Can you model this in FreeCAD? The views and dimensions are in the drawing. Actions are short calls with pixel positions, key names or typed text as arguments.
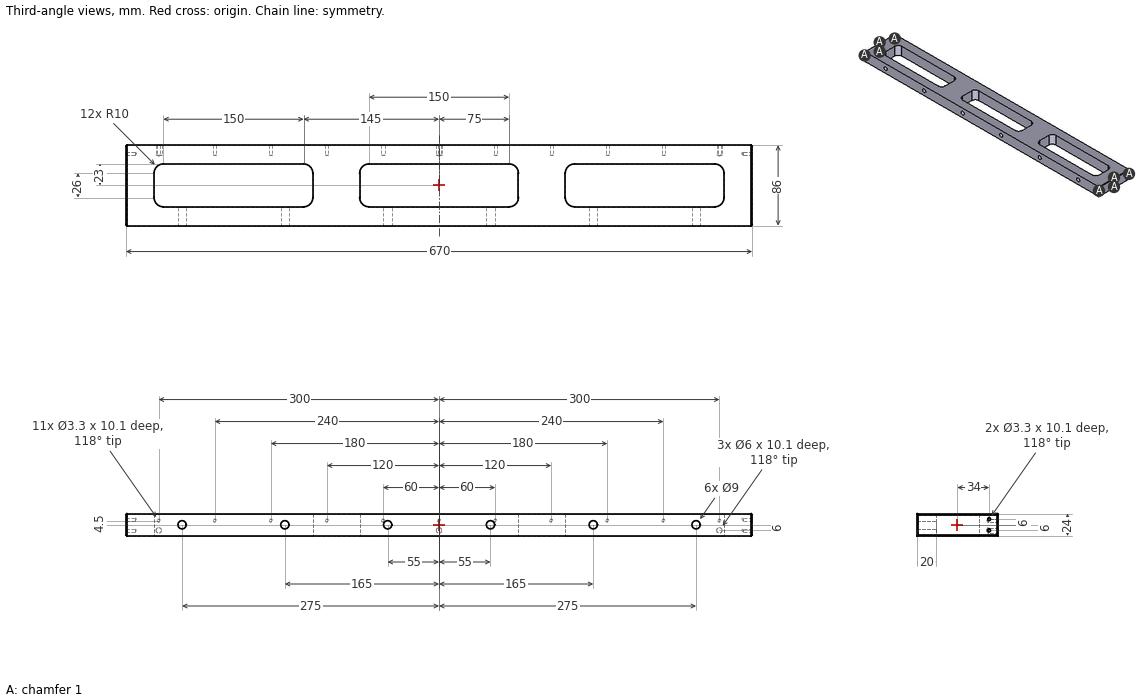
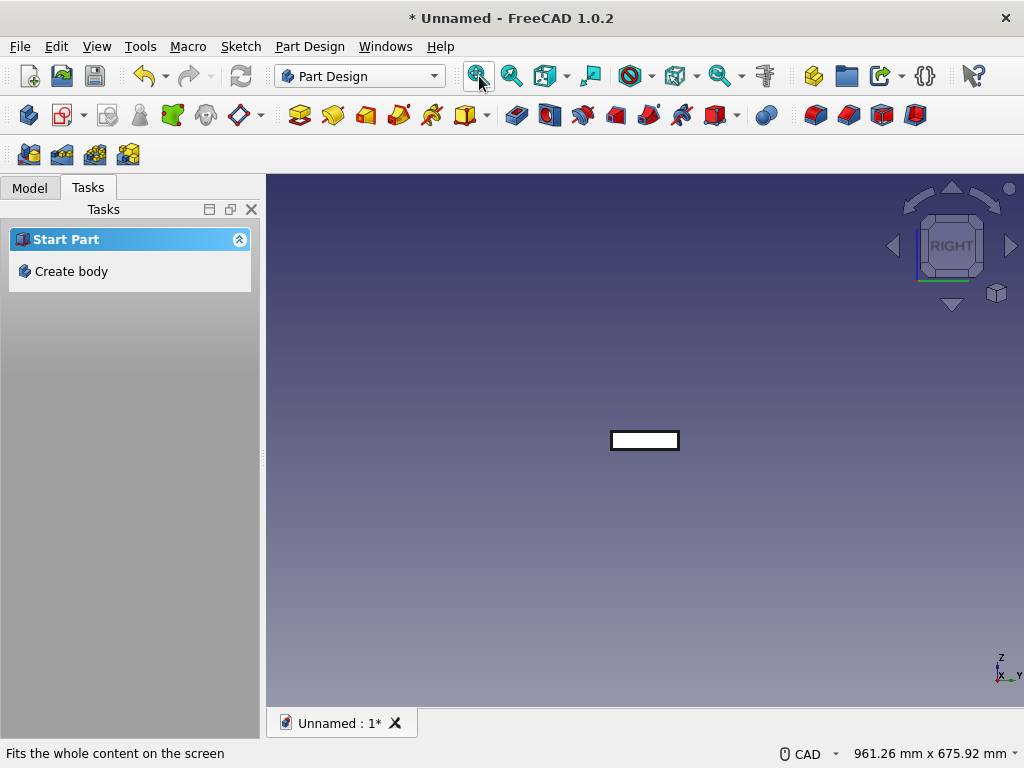
click(664, 439)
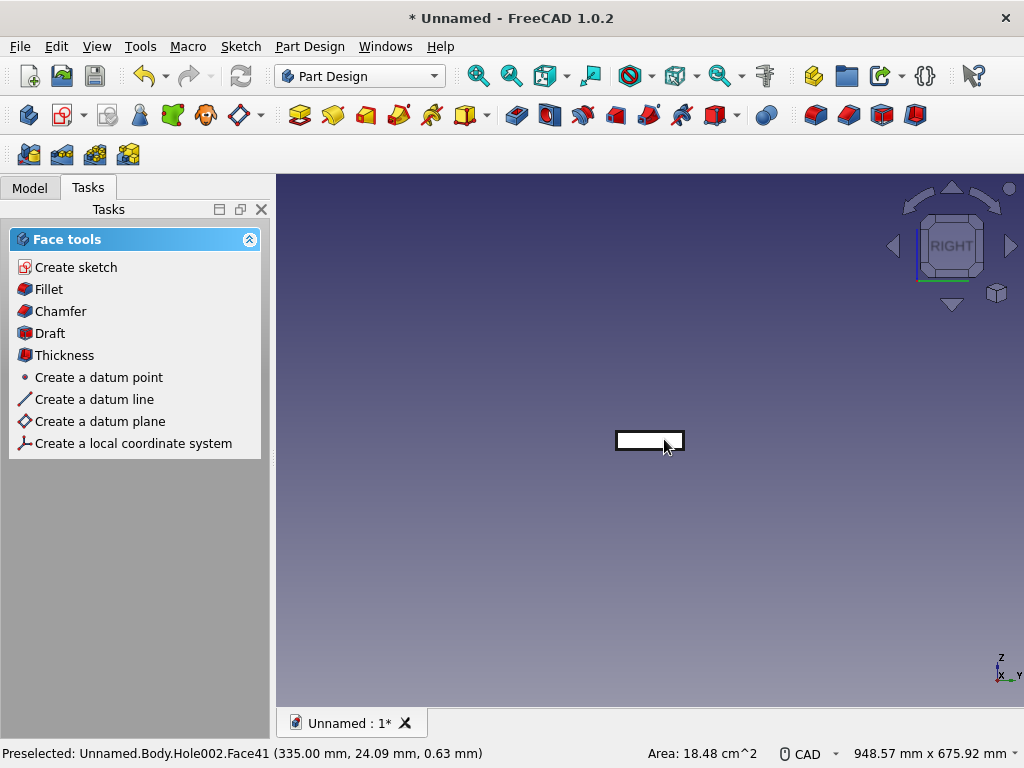
click(62, 116)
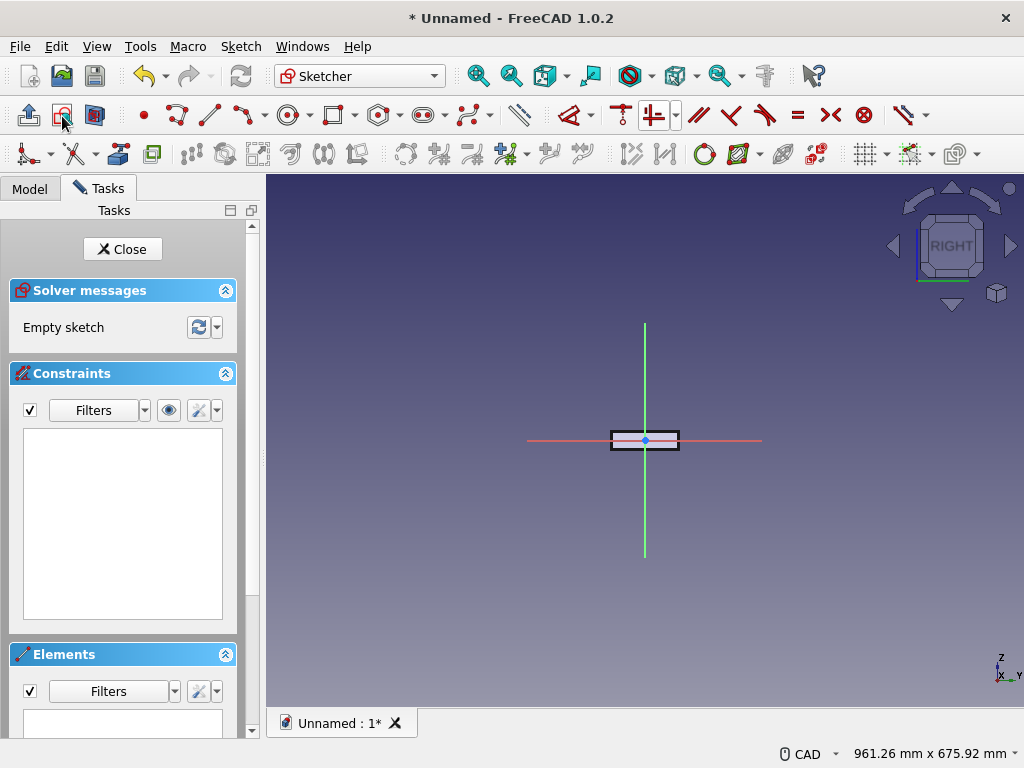
scroll(666, 440, up, 13)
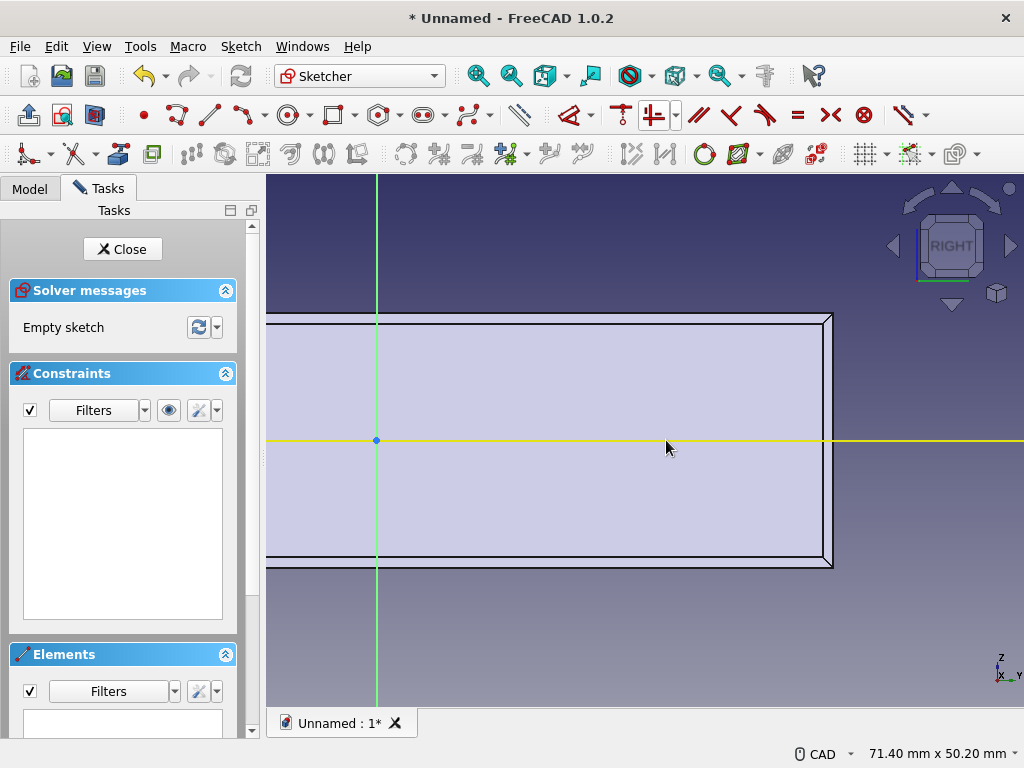
key(g)
key(c)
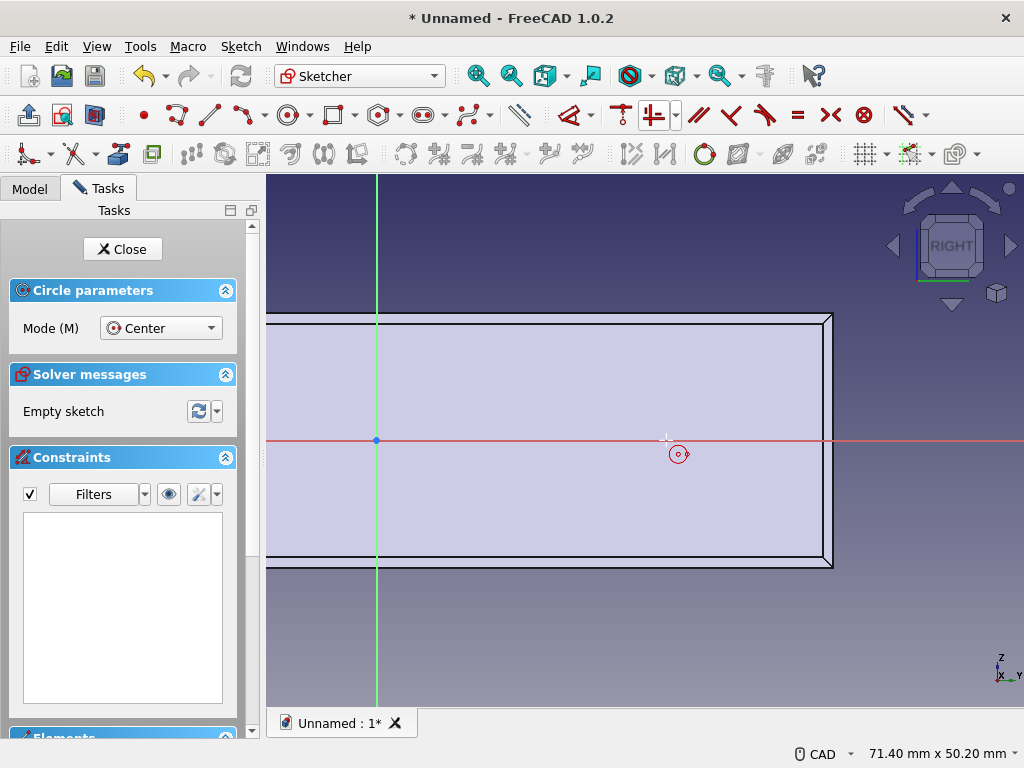
scroll(738, 377, up, 2)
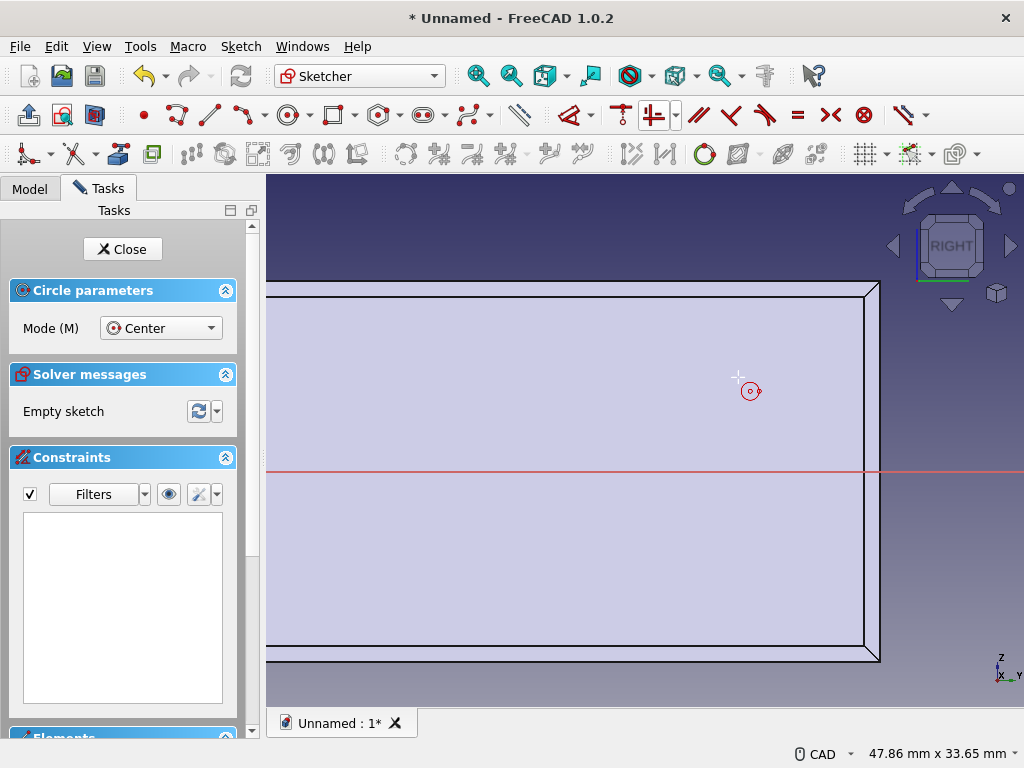
click(737, 377)
move(756, 358)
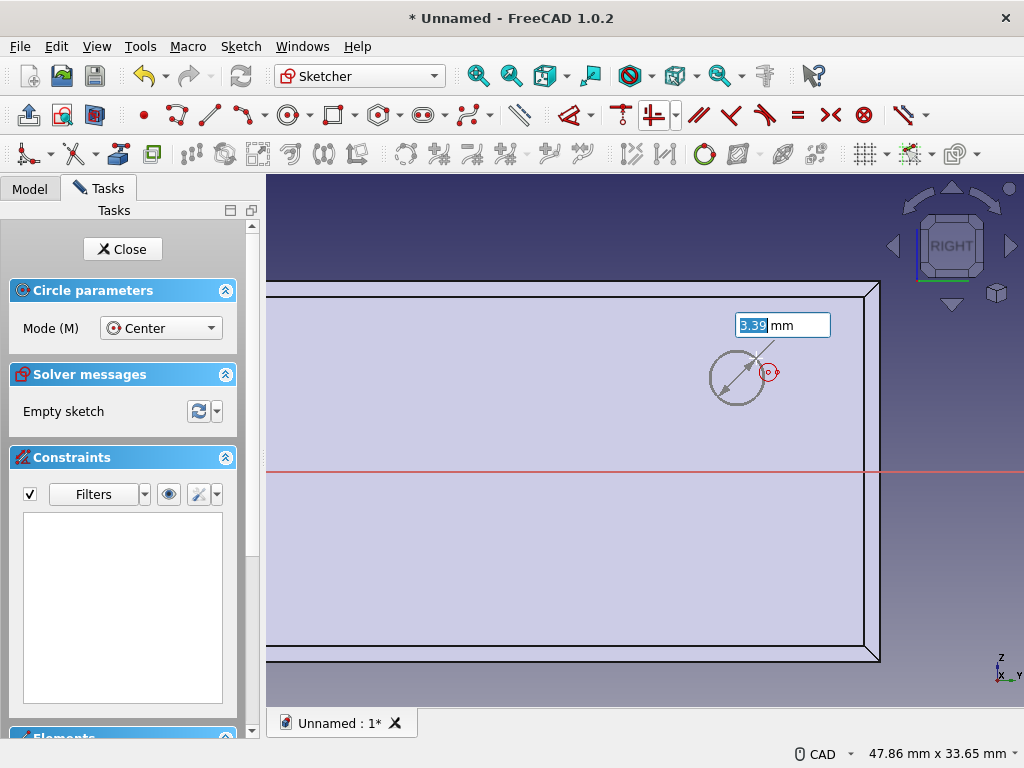
text(3.3)
key(Return)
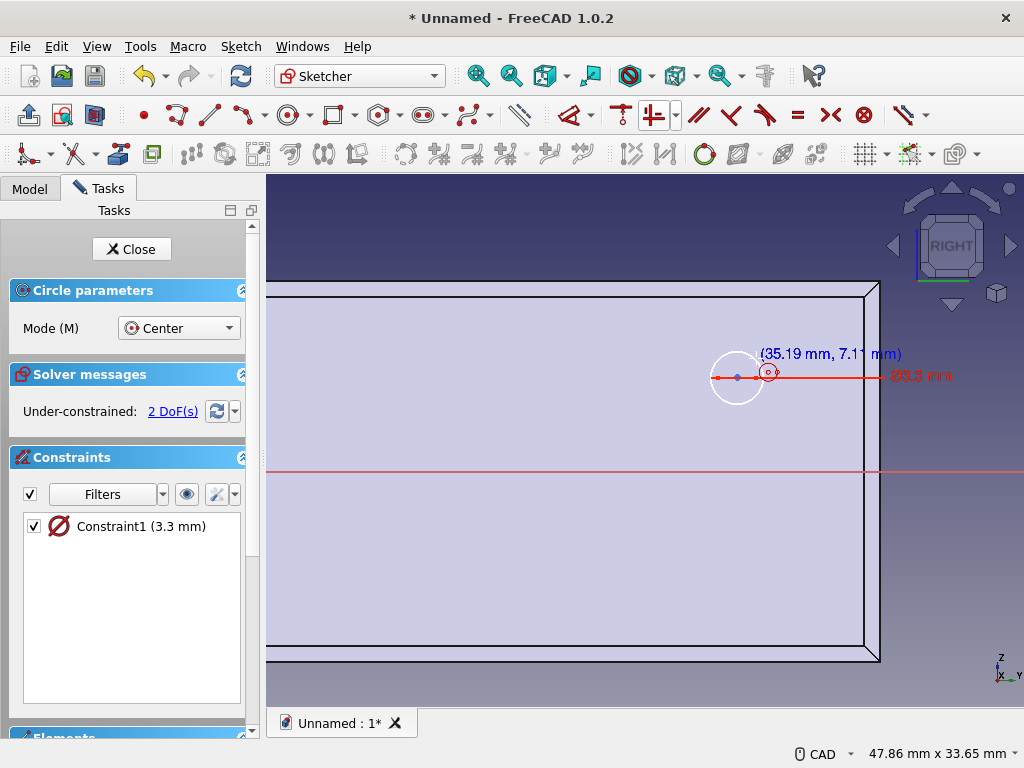
click(737, 567)
move(756, 548)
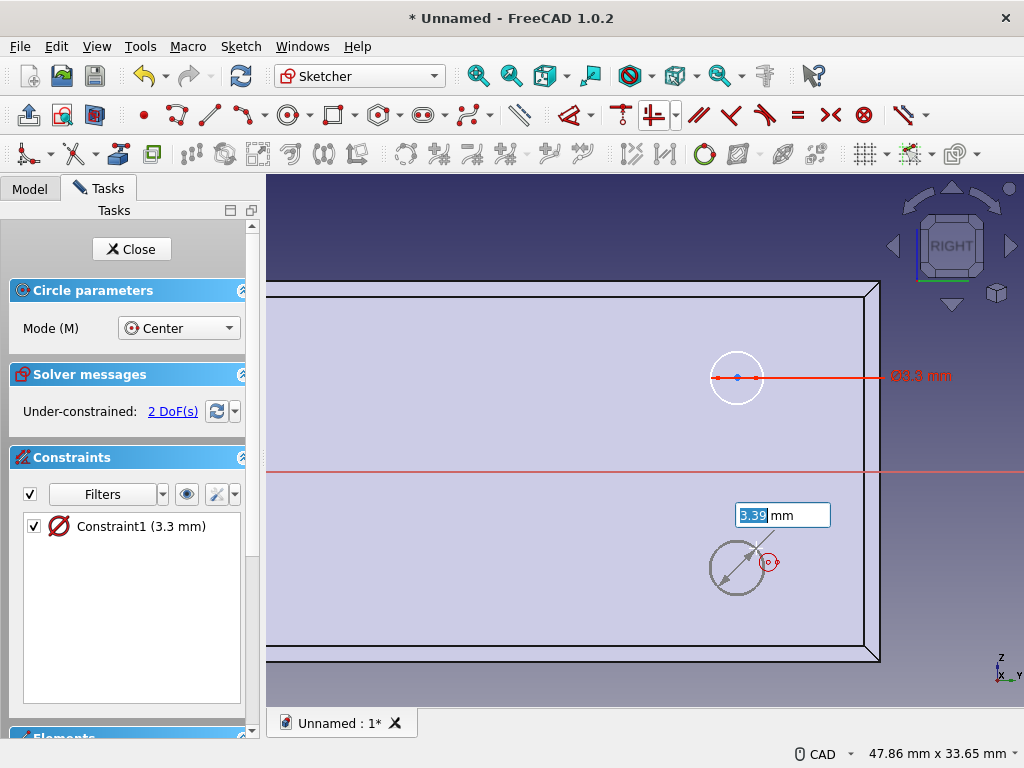
text(3.3)
key(Return)
key(Escape)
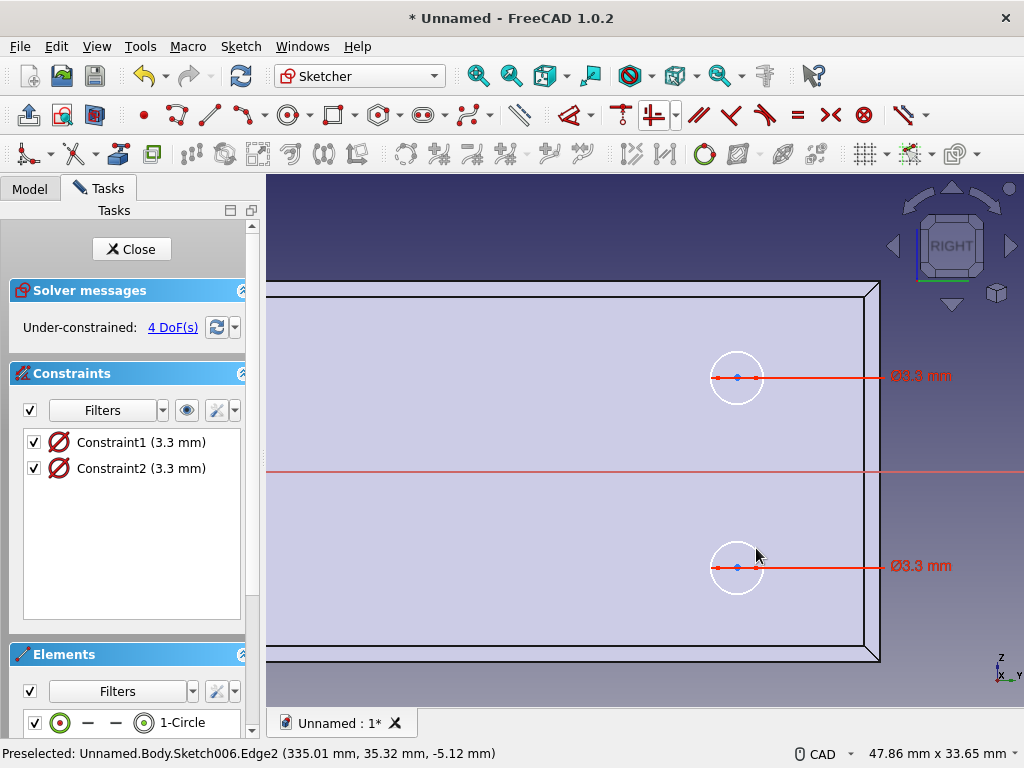
click(737, 378)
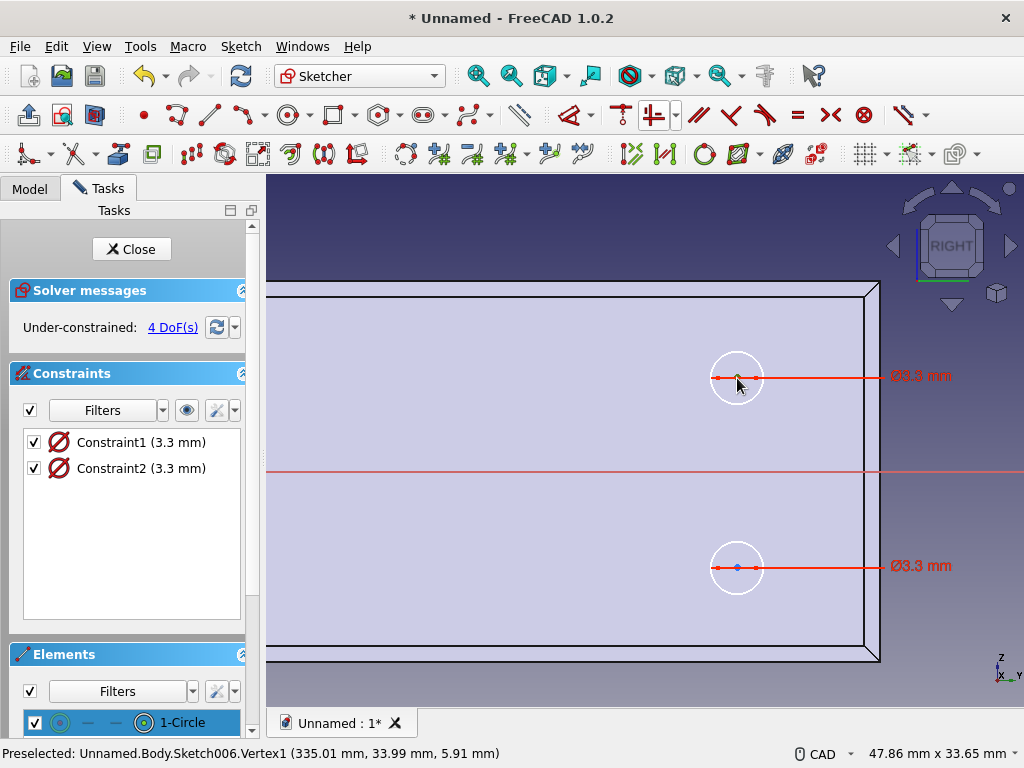
click(737, 568)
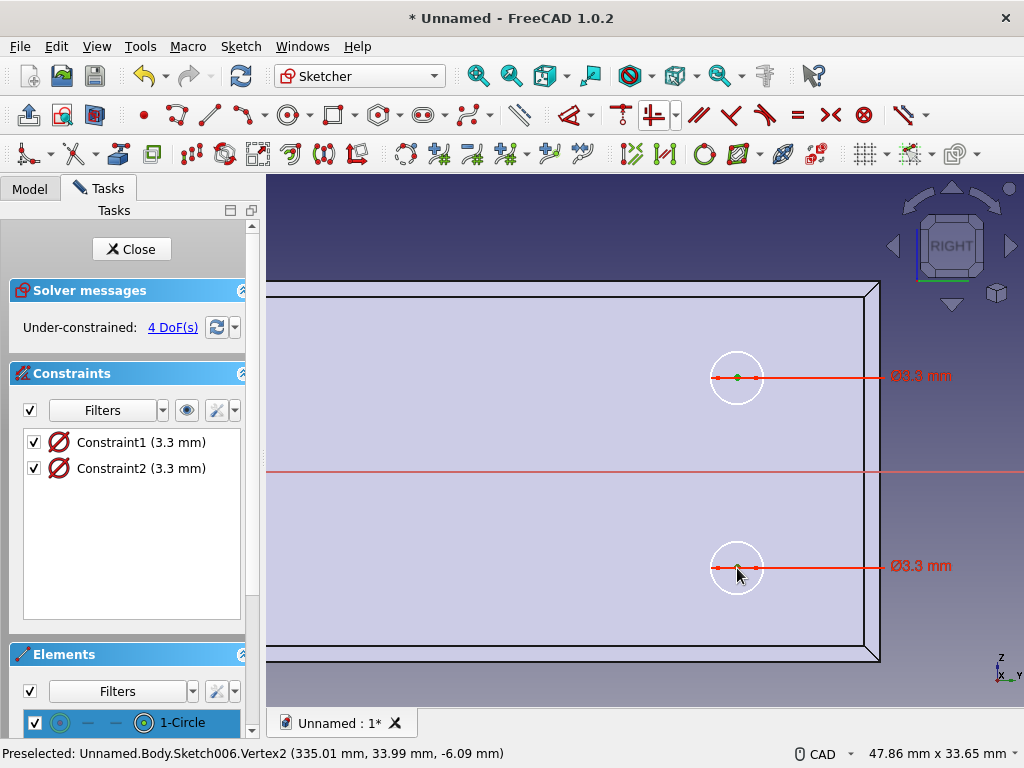
key(v)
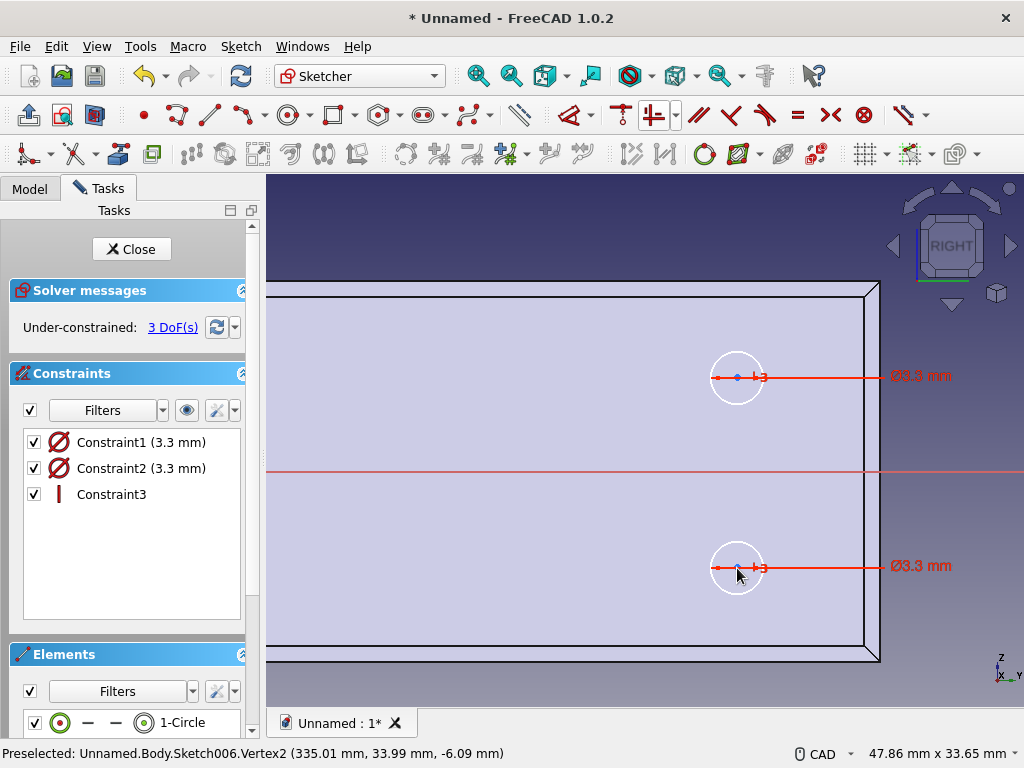
key(d)